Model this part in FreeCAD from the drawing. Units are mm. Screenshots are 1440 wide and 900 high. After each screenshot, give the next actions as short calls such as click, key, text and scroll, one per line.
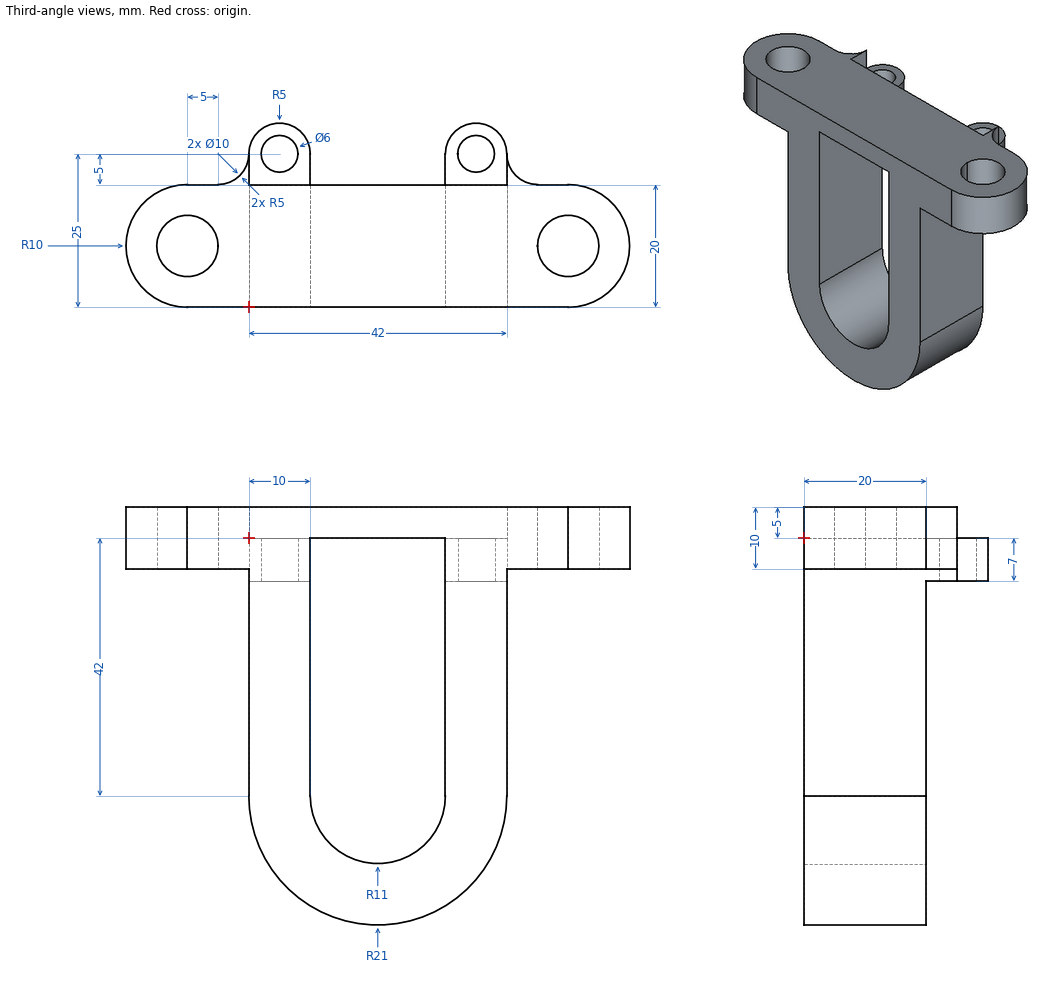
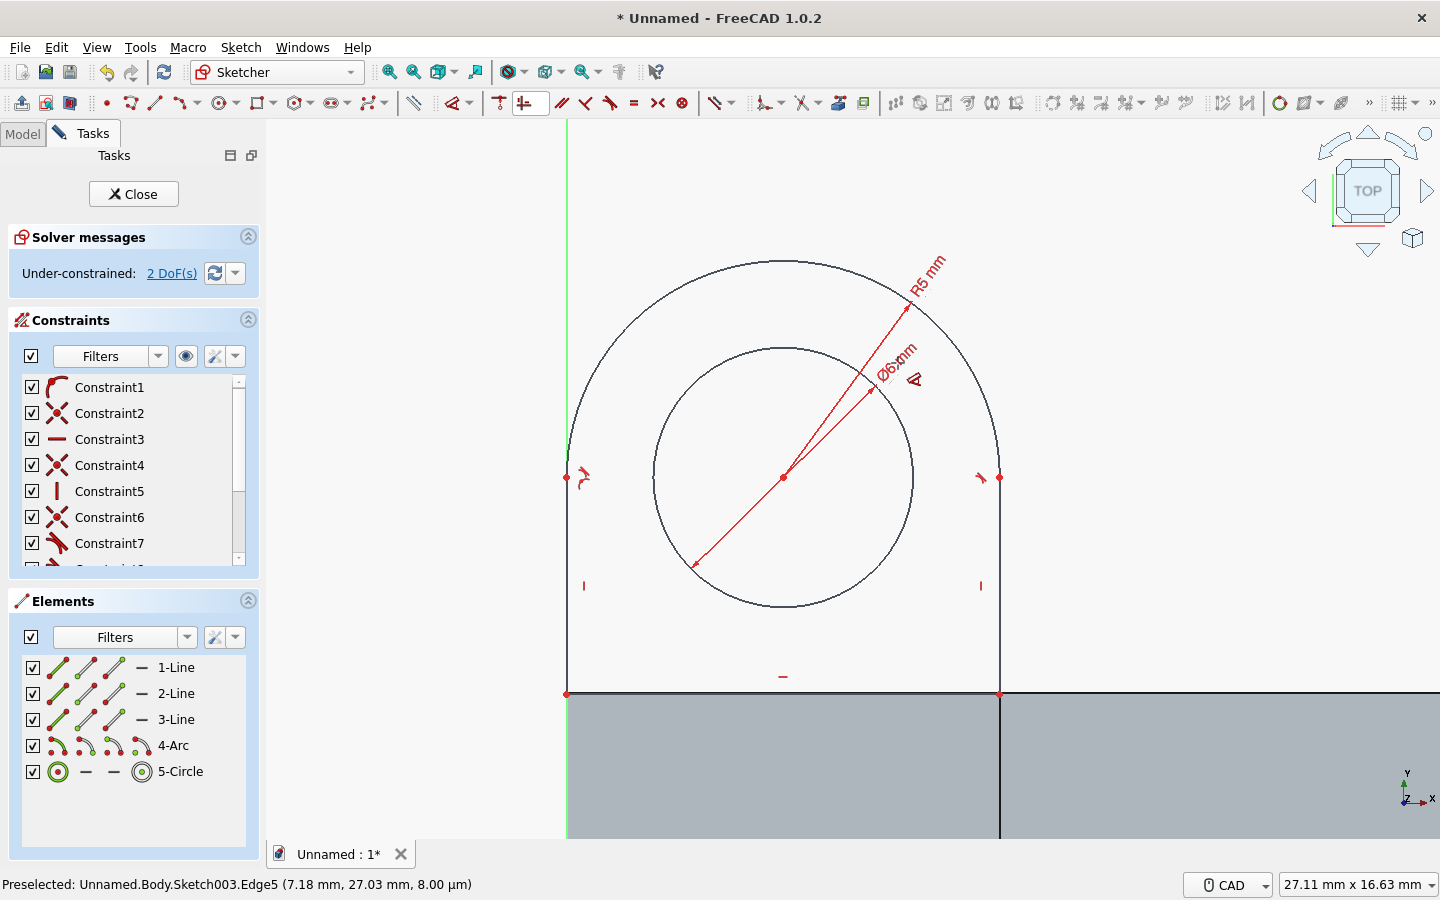
click(567, 542)
click(533, 586)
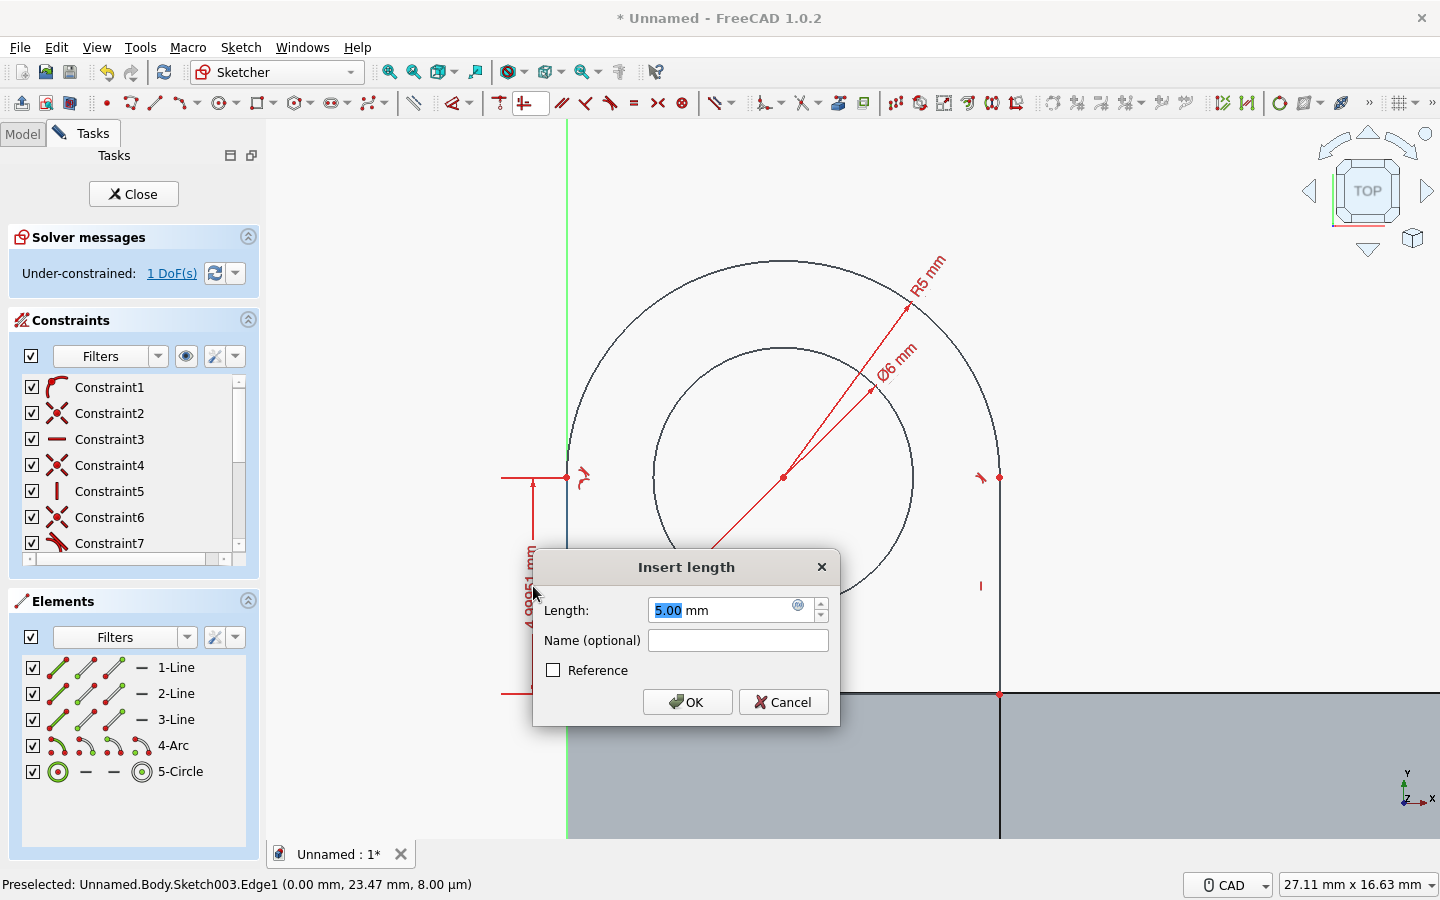
text(5)
key(Return)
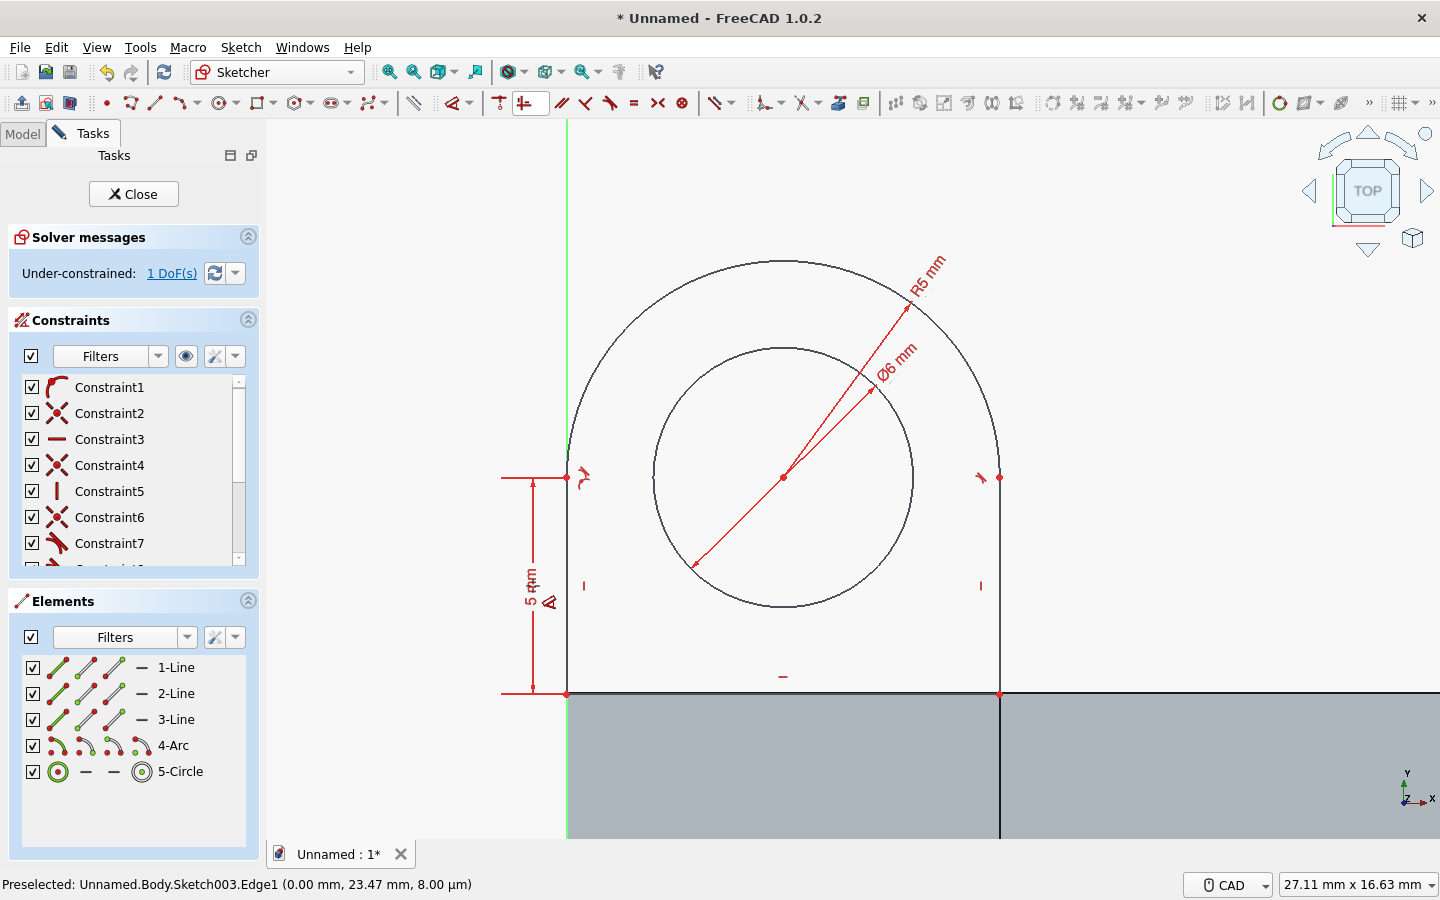
click(783, 478)
click(533, 644)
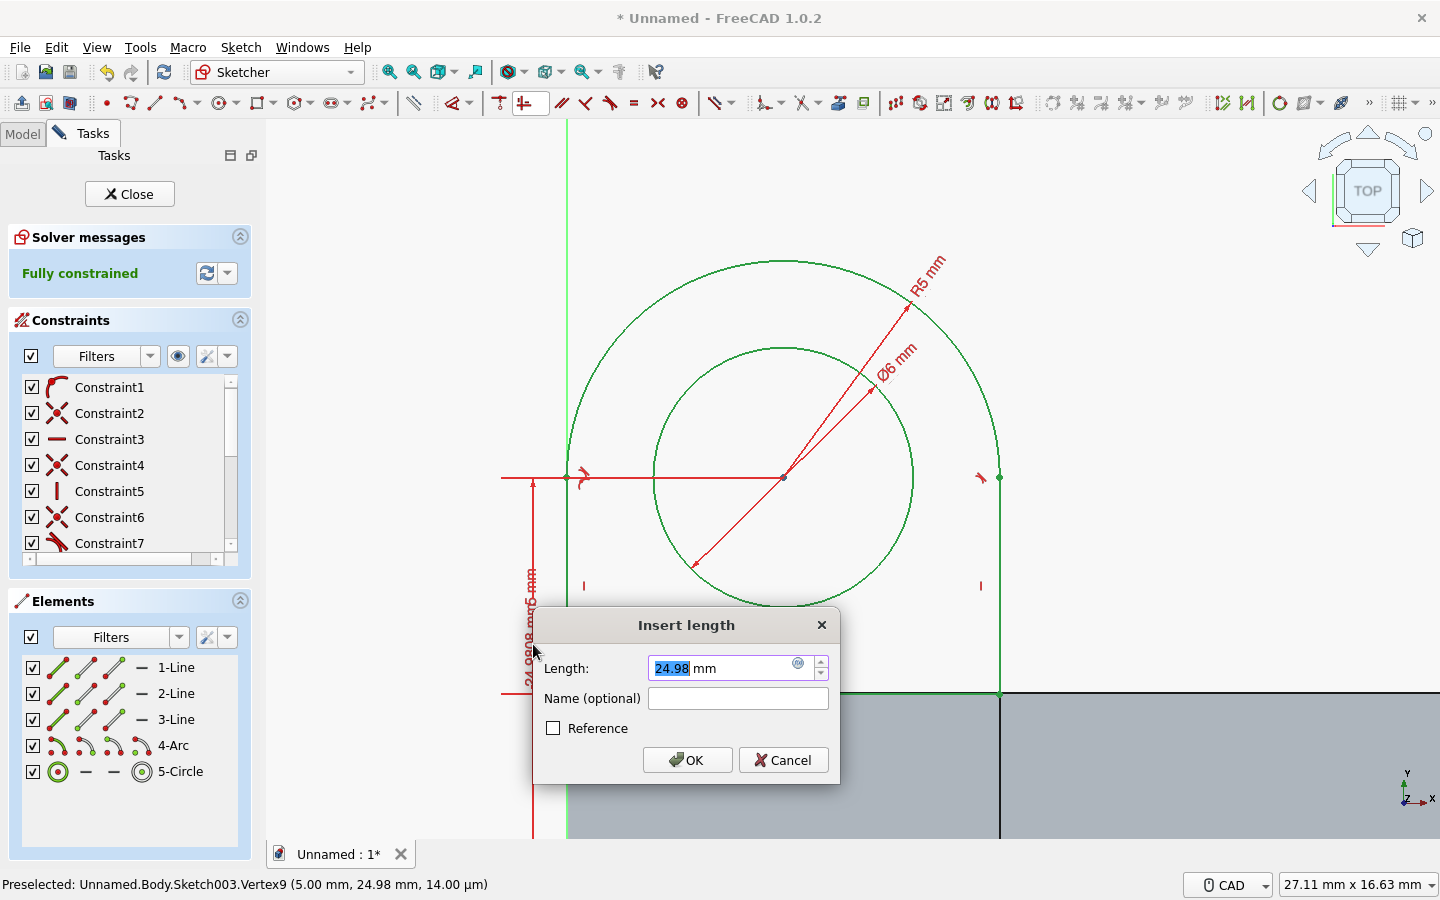
text(25)
key(Return)
key(Escape)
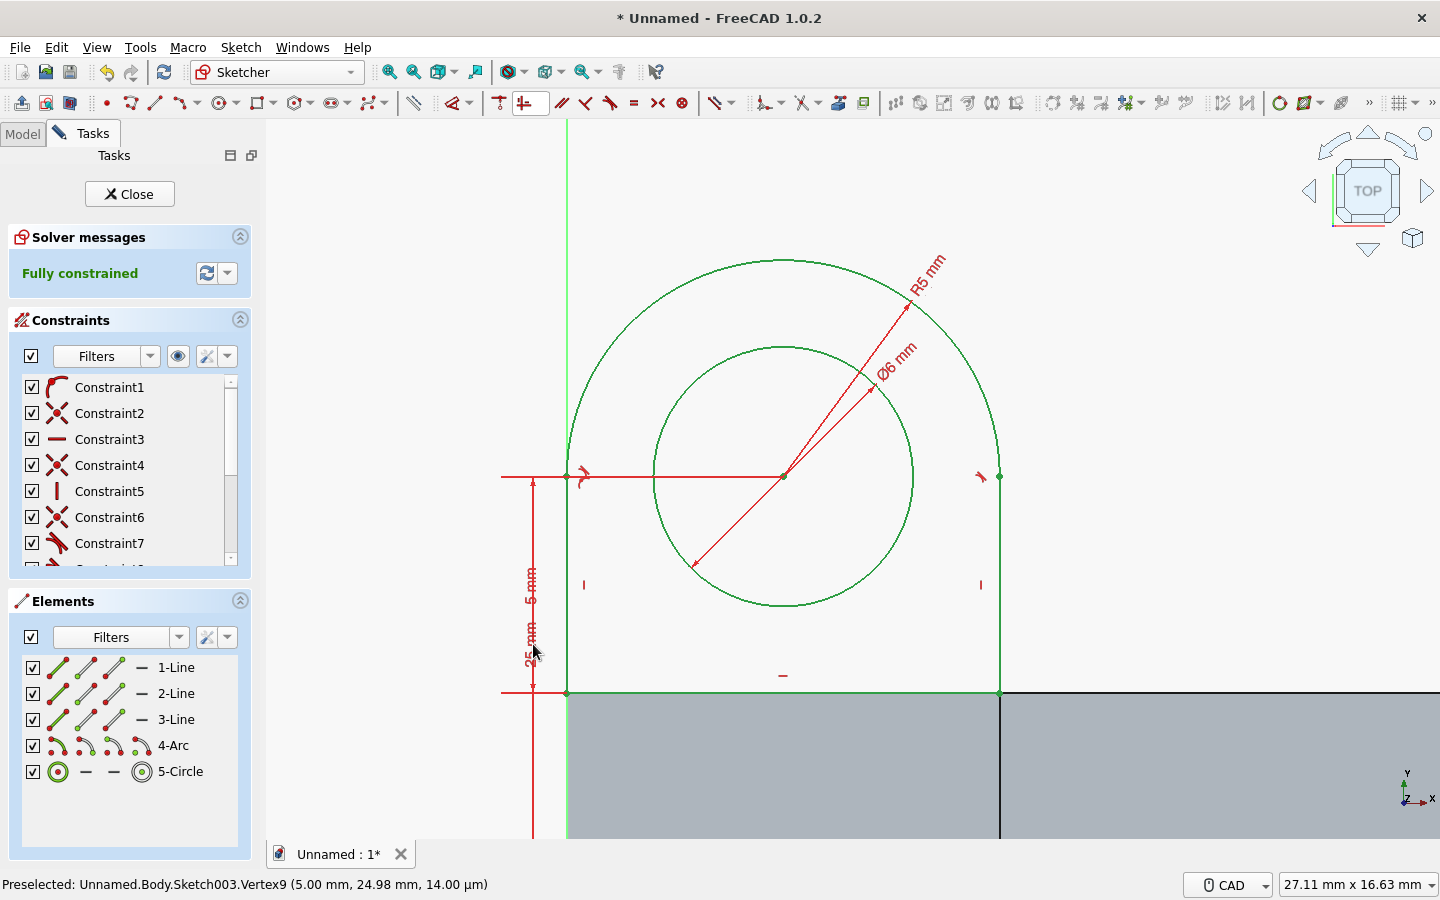
click(130, 194)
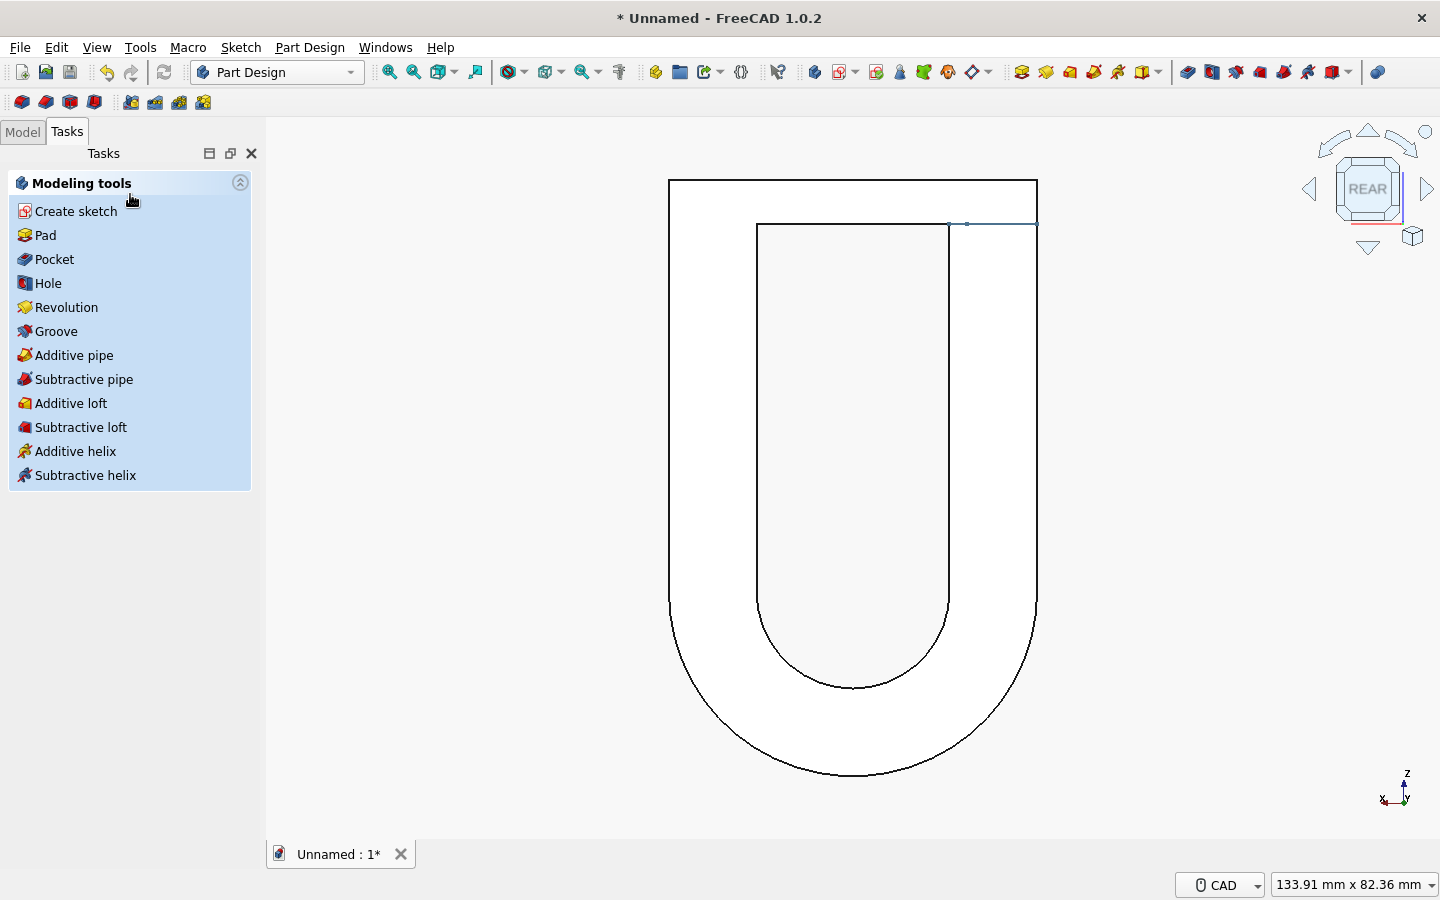
click(1022, 72)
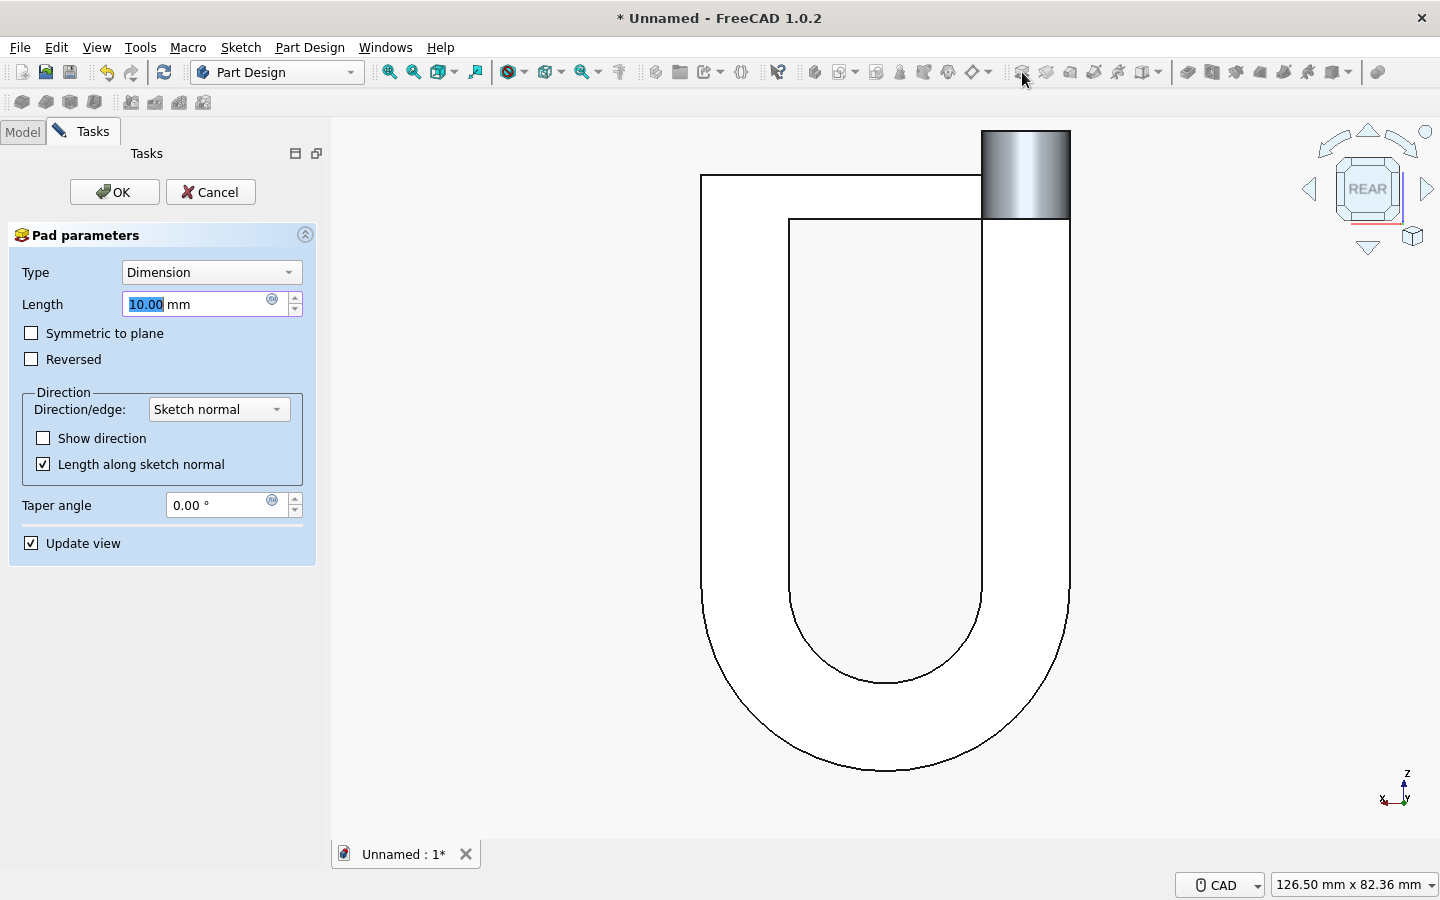
text(7)
key(Tab)